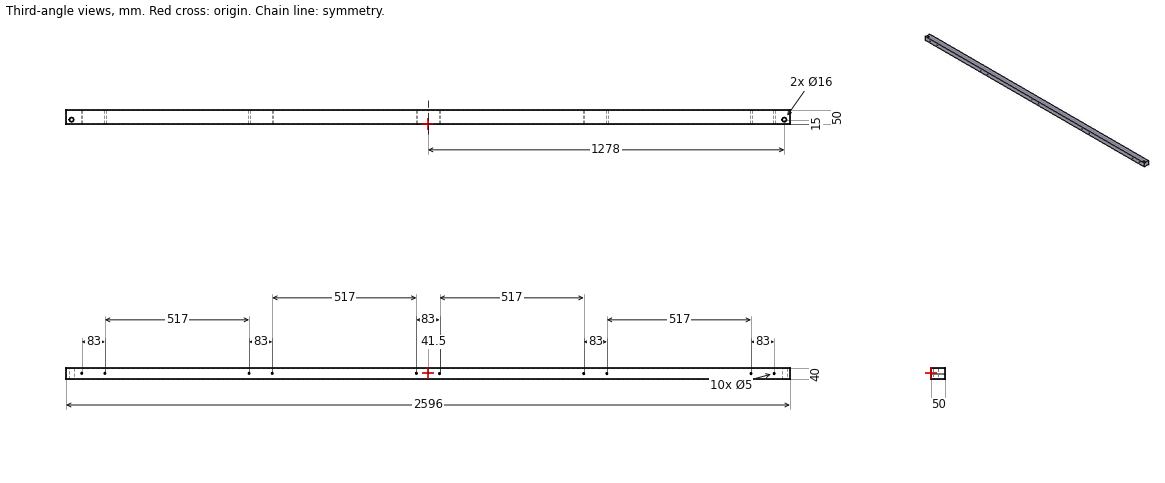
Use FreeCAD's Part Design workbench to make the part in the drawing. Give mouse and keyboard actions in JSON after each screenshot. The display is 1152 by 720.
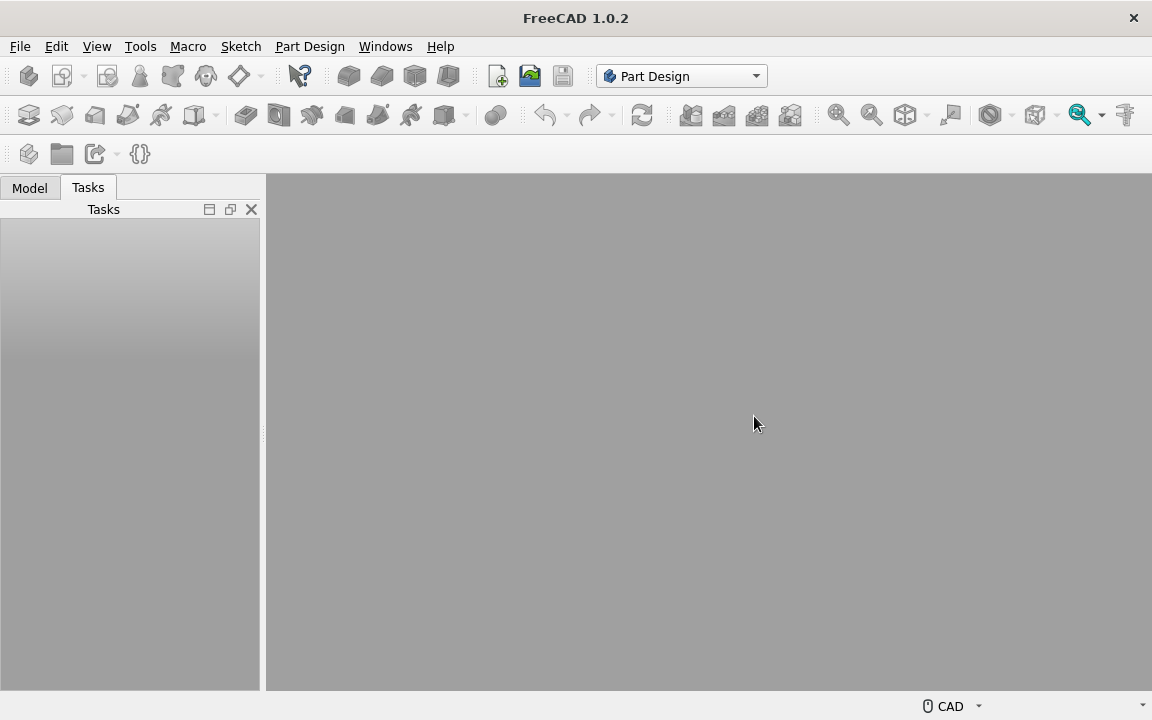
{"action": "left_click", "coordinate": [497, 76]}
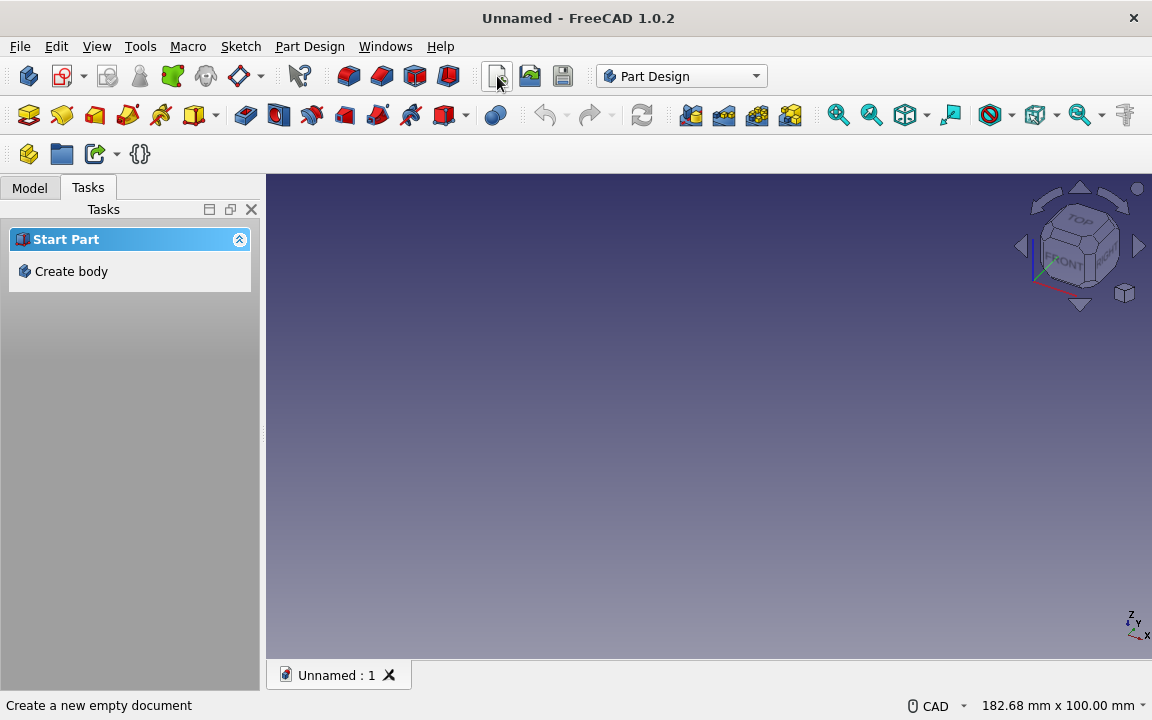
{"action": "left_click", "coordinate": [62, 76]}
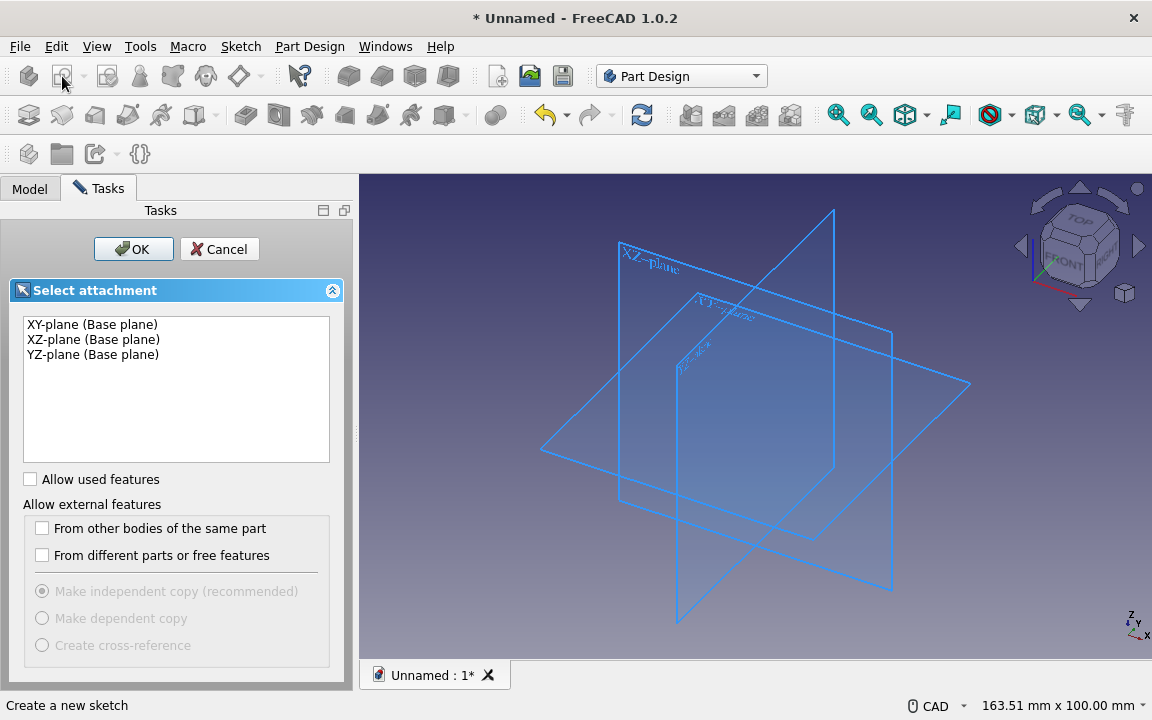
{"action": "left_click", "coordinate": [84, 340]}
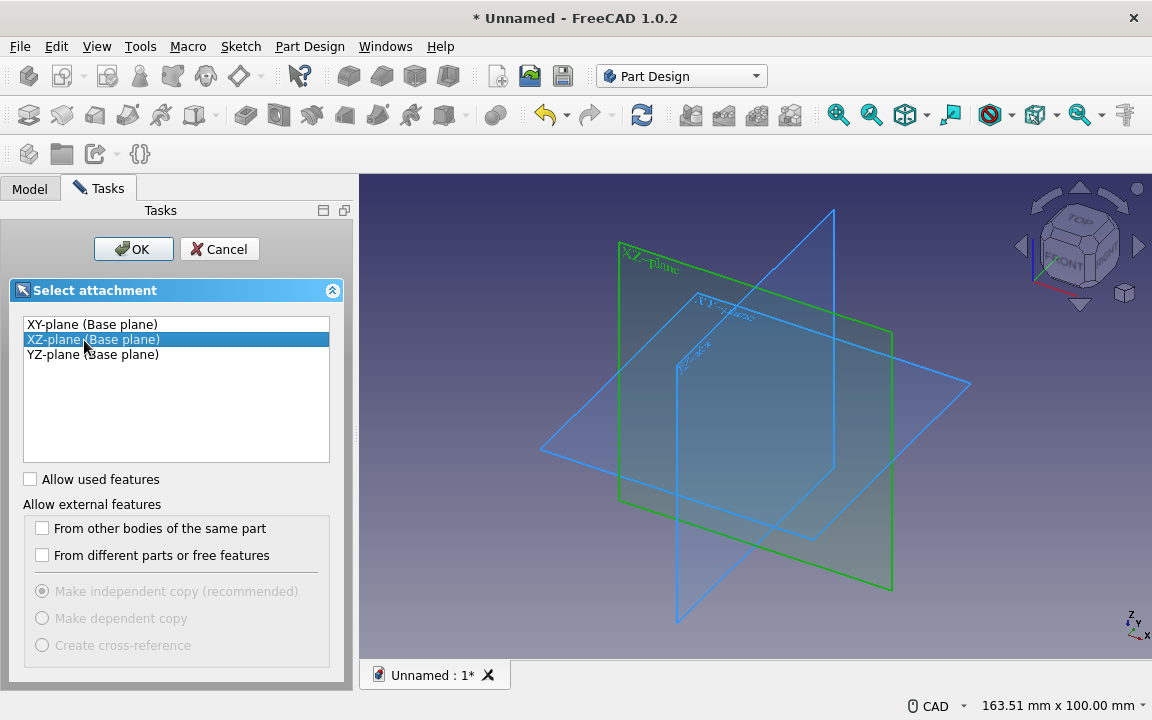
{"action": "left_click", "coordinate": [134, 249]}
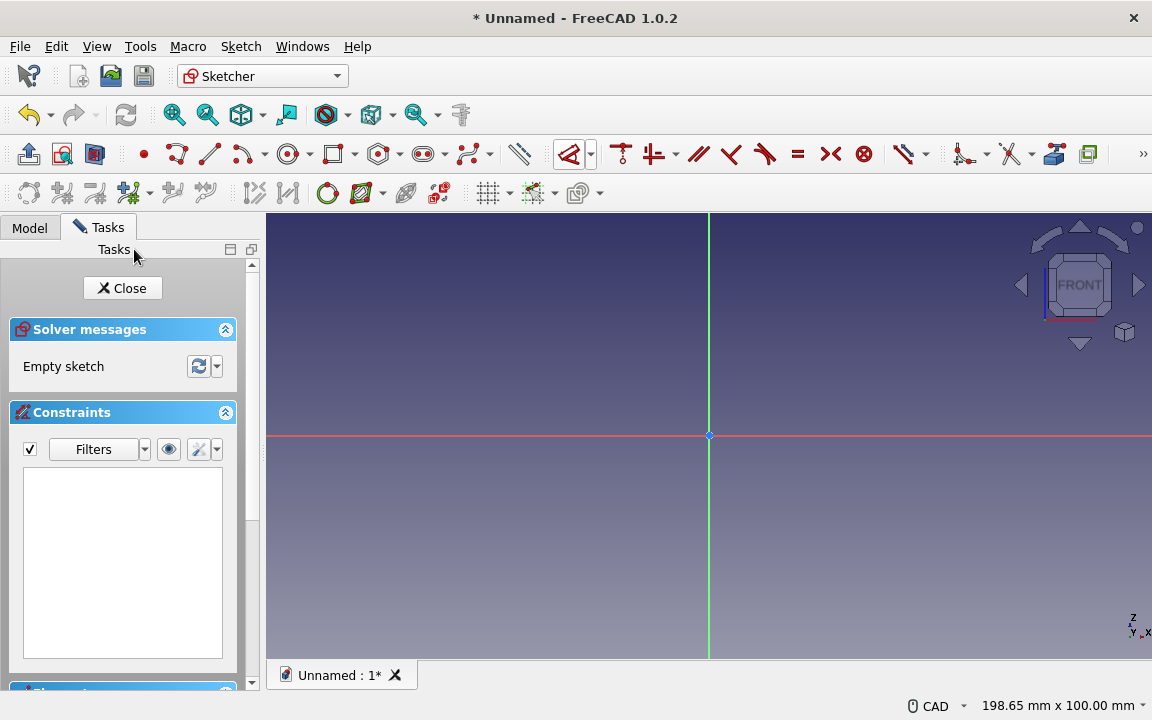
{"action": "scroll", "coordinate": [637, 436], "scroll_direction": "down", "scroll_amount": 15}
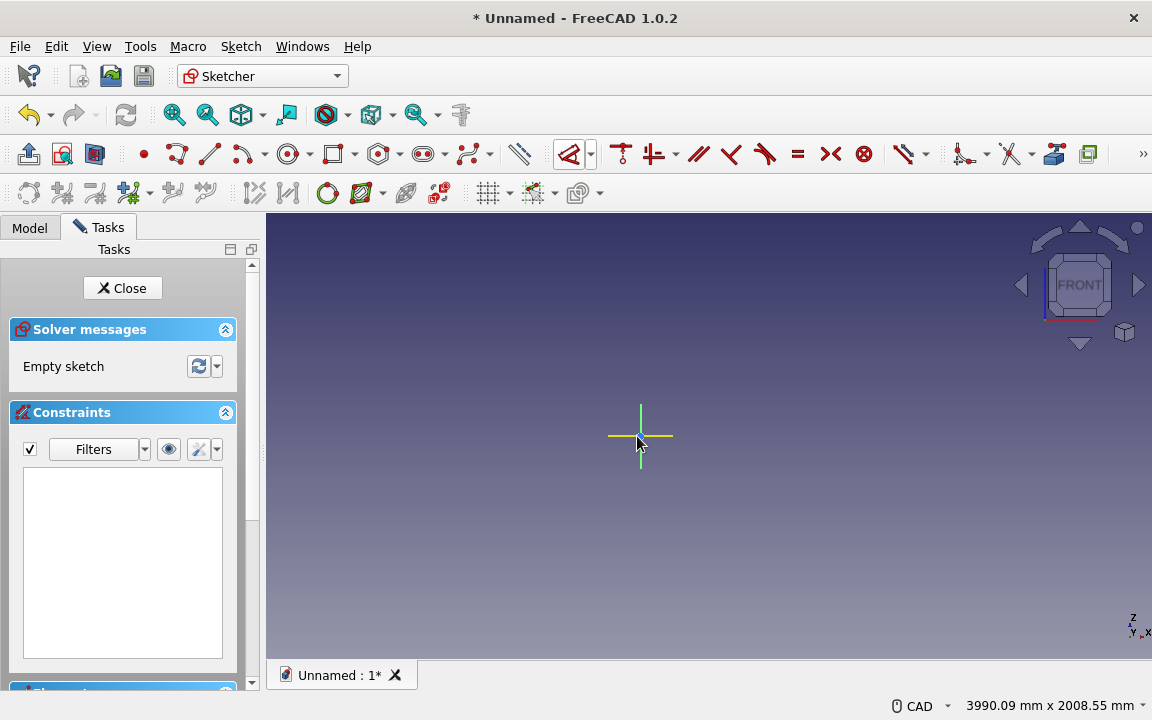
{"action": "left_click", "coordinate": [354, 154]}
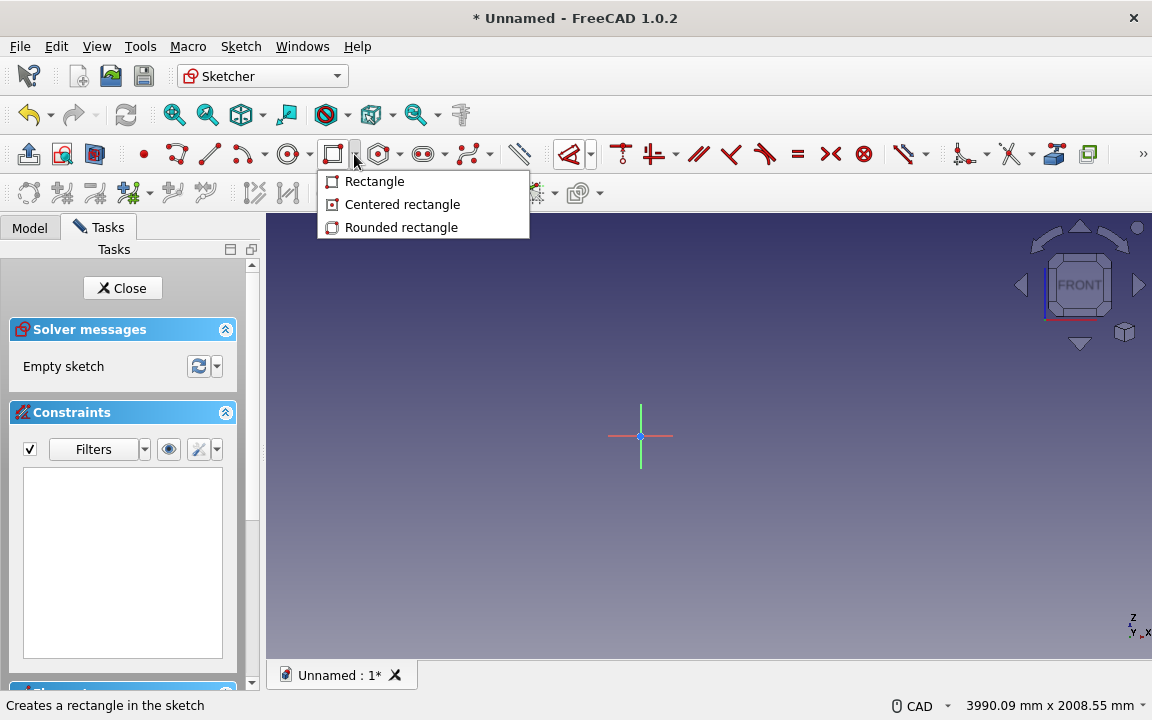
{"action": "left_click", "coordinate": [424, 204]}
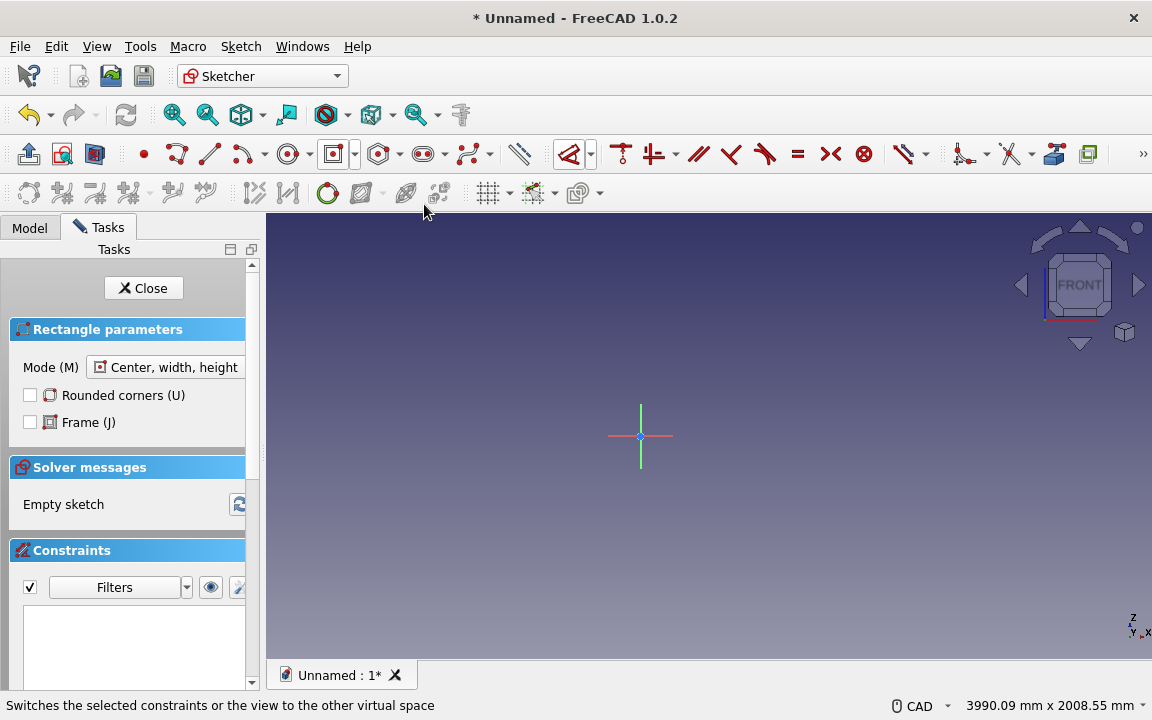
{"action": "scroll", "coordinate": [641, 436], "scroll_direction": "up", "scroll_amount": 7}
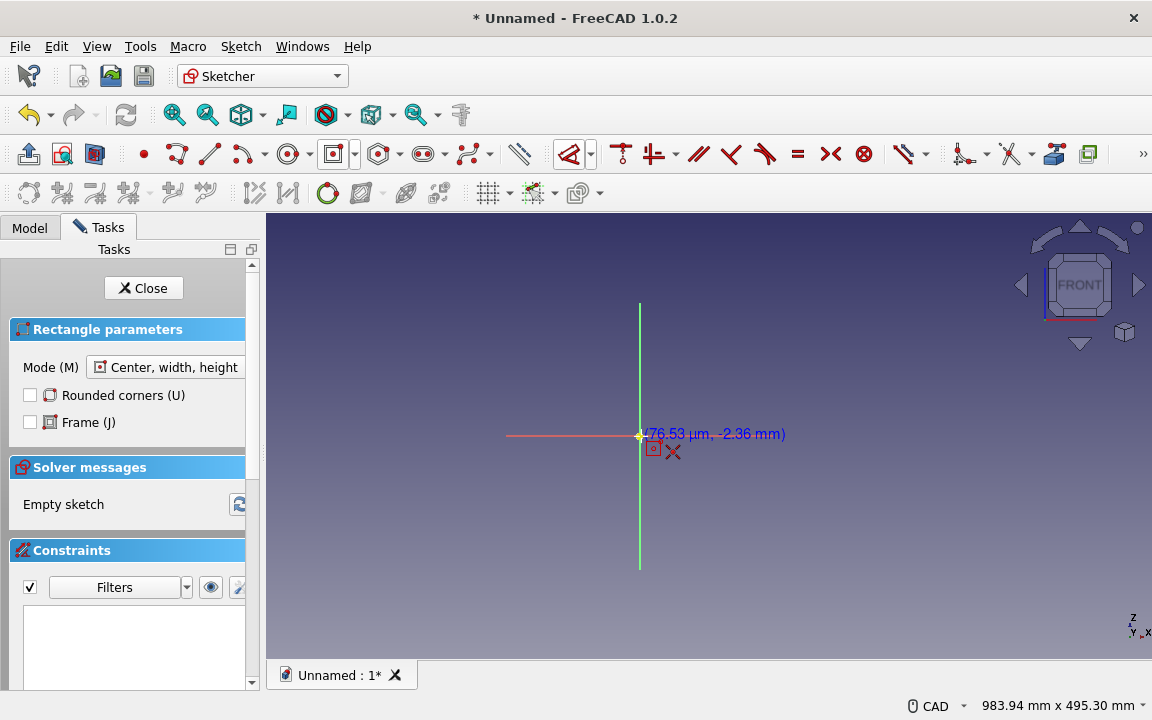
{"action": "scroll", "coordinate": [641, 436], "scroll_direction": "down", "scroll_amount": 8}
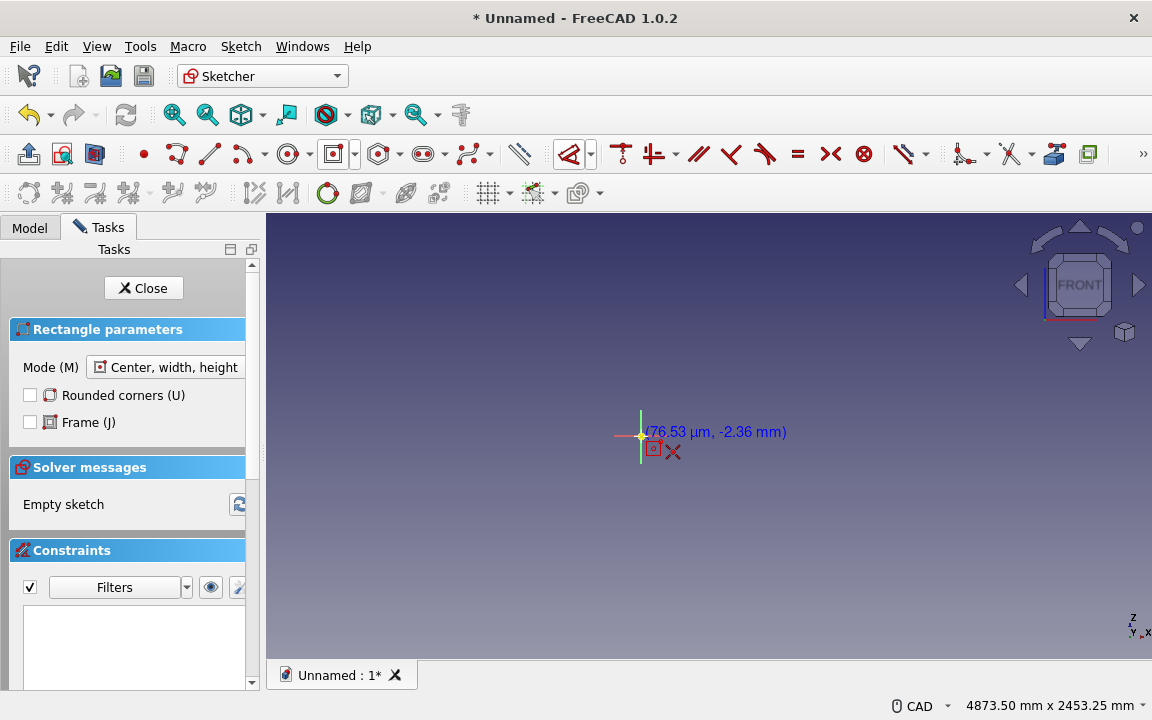
{"action": "left_click", "coordinate": [641, 436]}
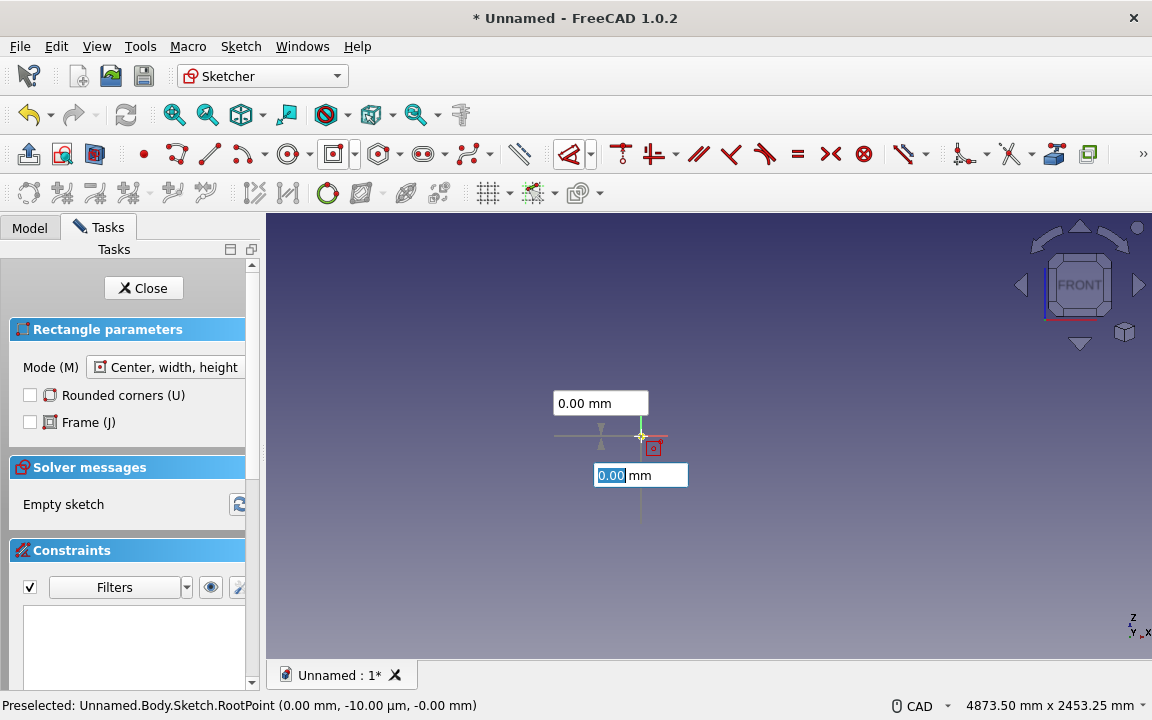
{"action": "scroll", "coordinate": [877, 433], "scroll_direction": "up", "scroll_amount": 8}
{"action": "mouse_move", "coordinate": [874, 430]}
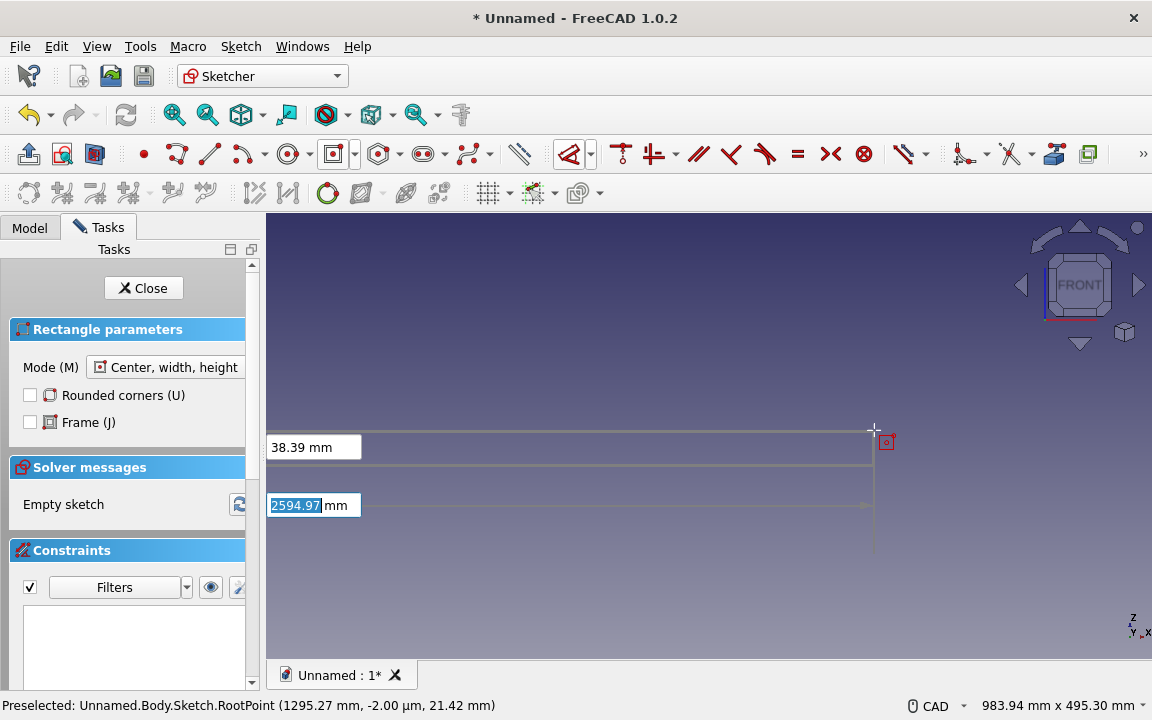
{"action": "type", "text": "2596"}
{"action": "key", "text": "Tab"}
{"action": "type", "text": "40"}
{"action": "key", "text": "Return"}
{"action": "key", "text": "Escape"}